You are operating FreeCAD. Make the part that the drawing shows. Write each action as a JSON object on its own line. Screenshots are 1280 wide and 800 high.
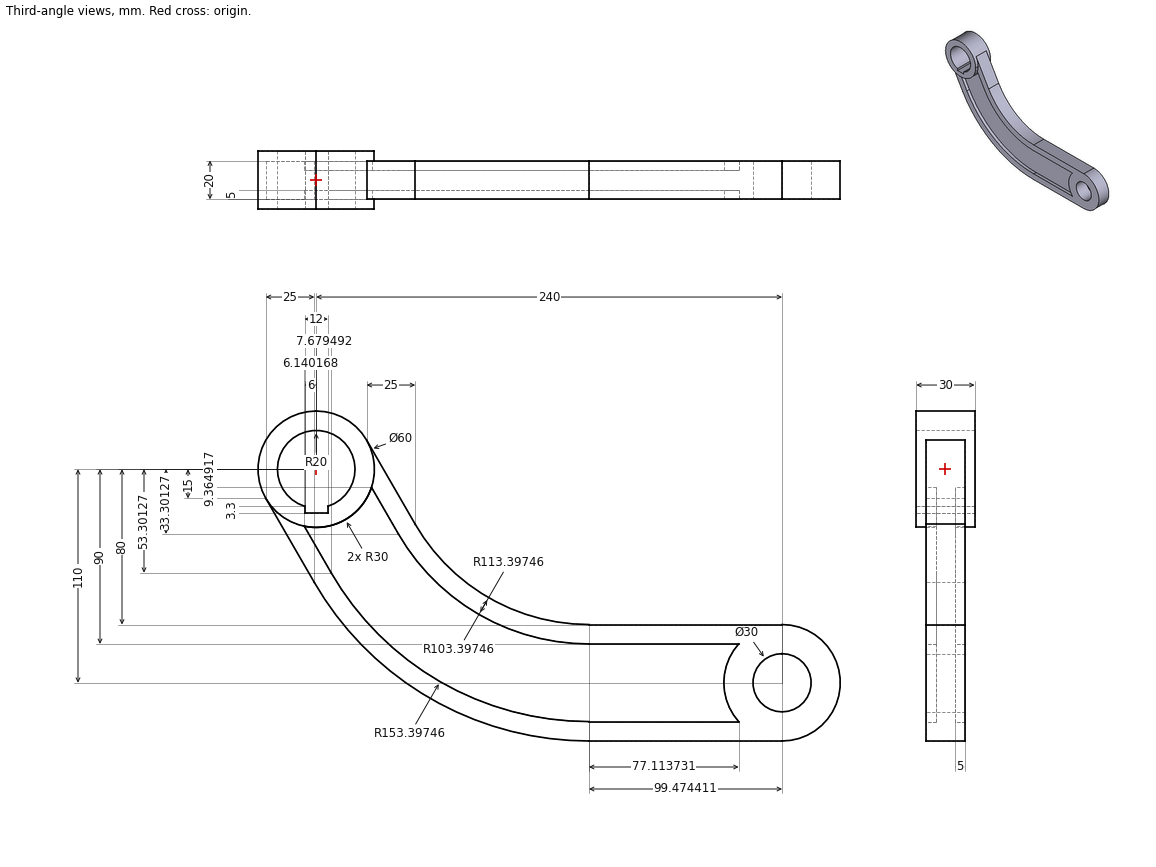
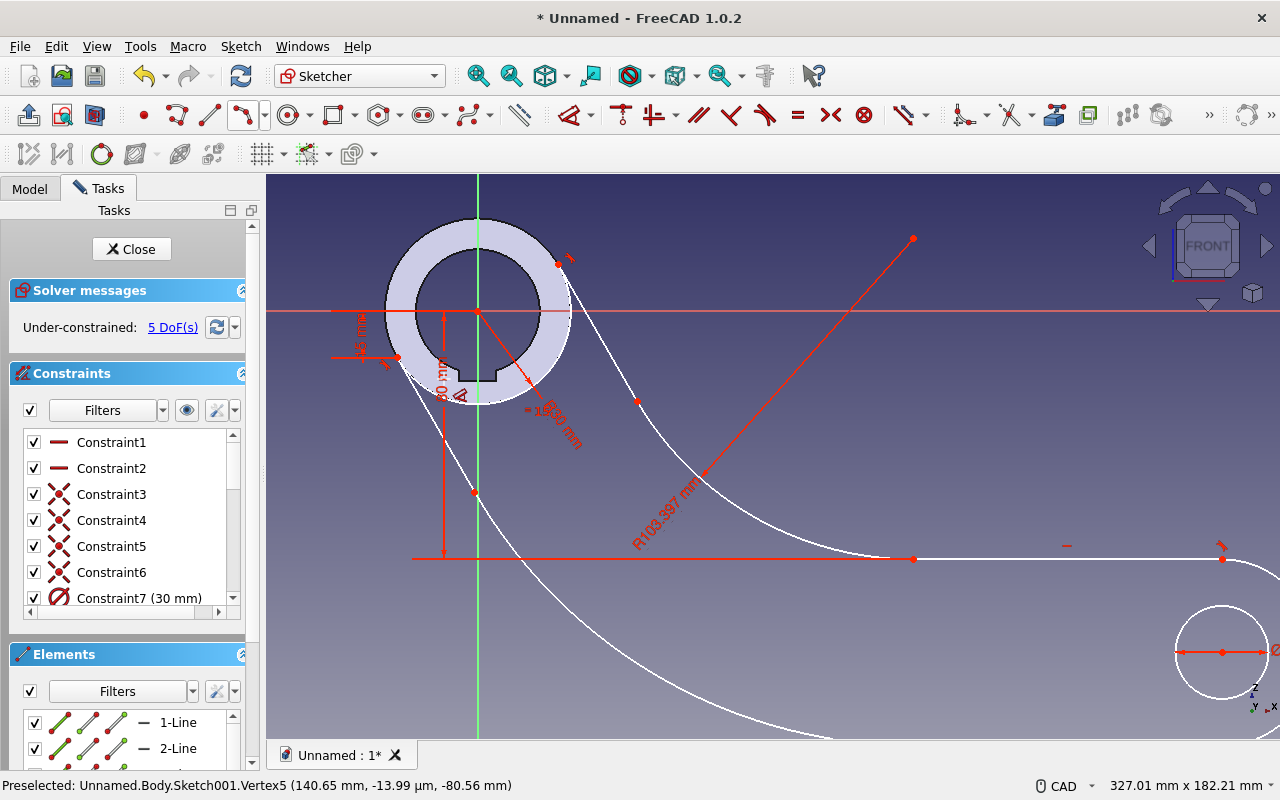
{"action": "left_click", "coordinate": [452, 452]}
{"action": "left_click", "coordinate": [436, 526]}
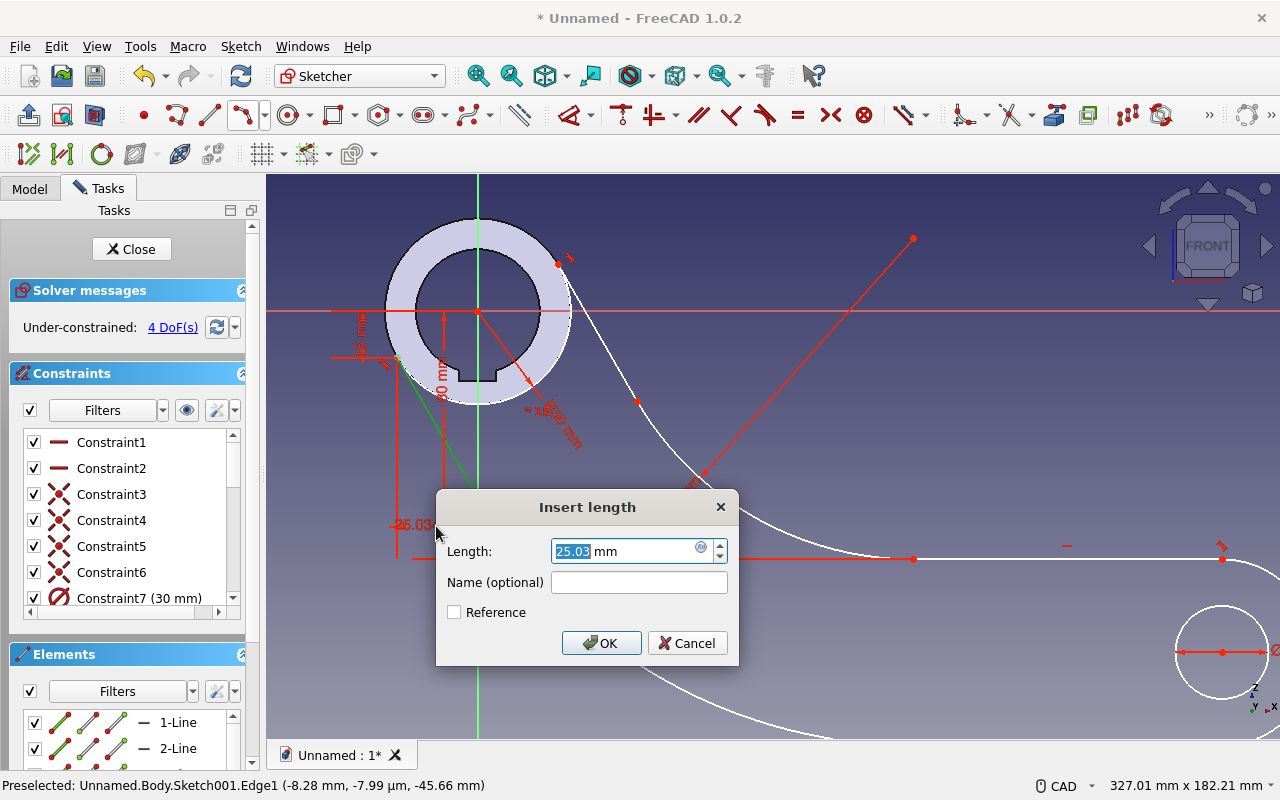
{"action": "type", "text": "25"}
{"action": "key", "text": "Return"}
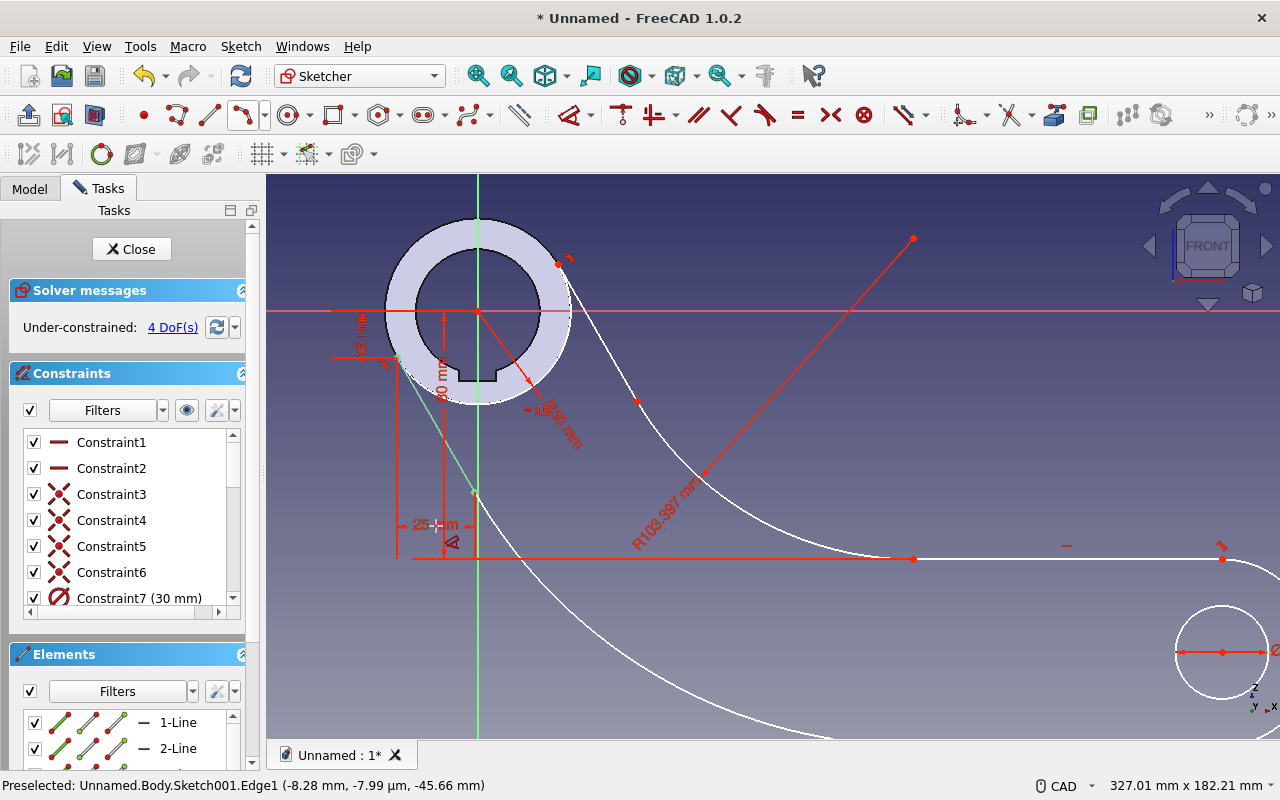
{"action": "left_click", "coordinate": [614, 360]}
{"action": "left_click", "coordinate": [598, 231]}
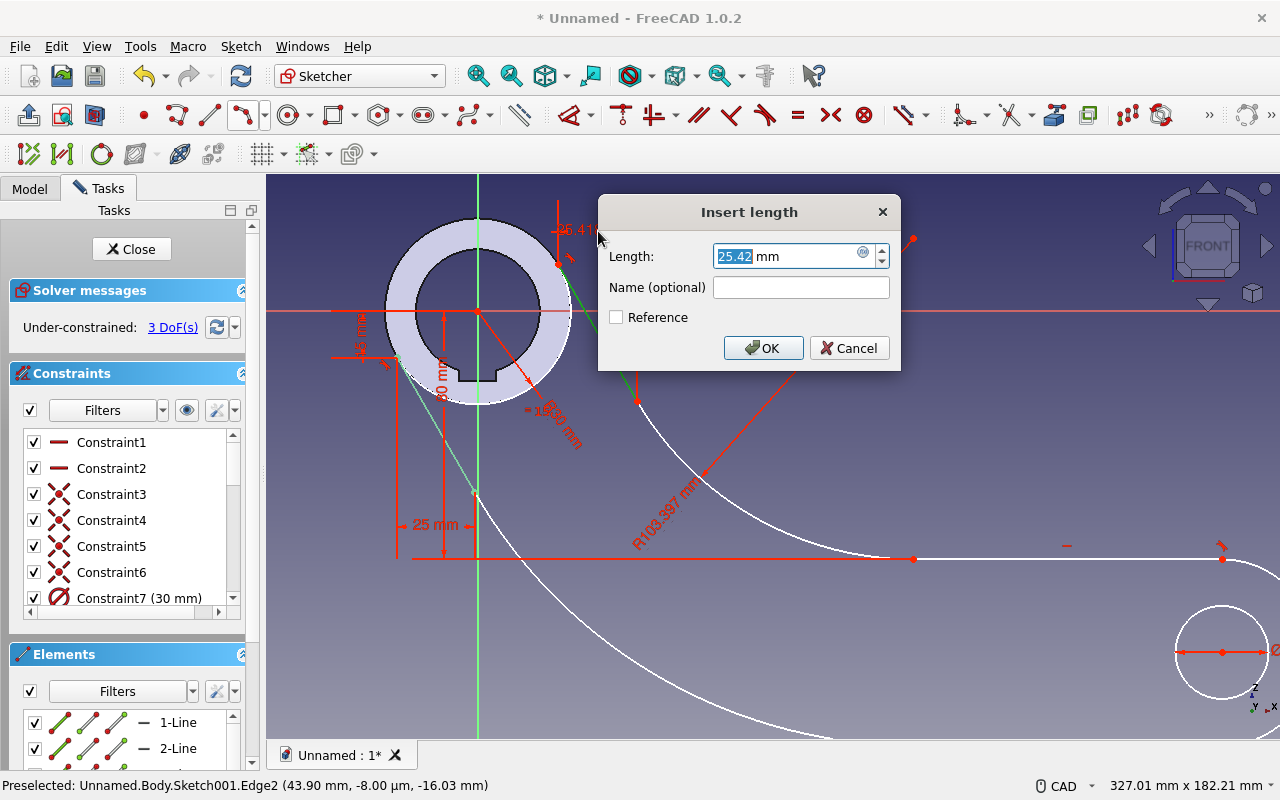
{"action": "type", "text": "25"}
{"action": "key", "text": "Return"}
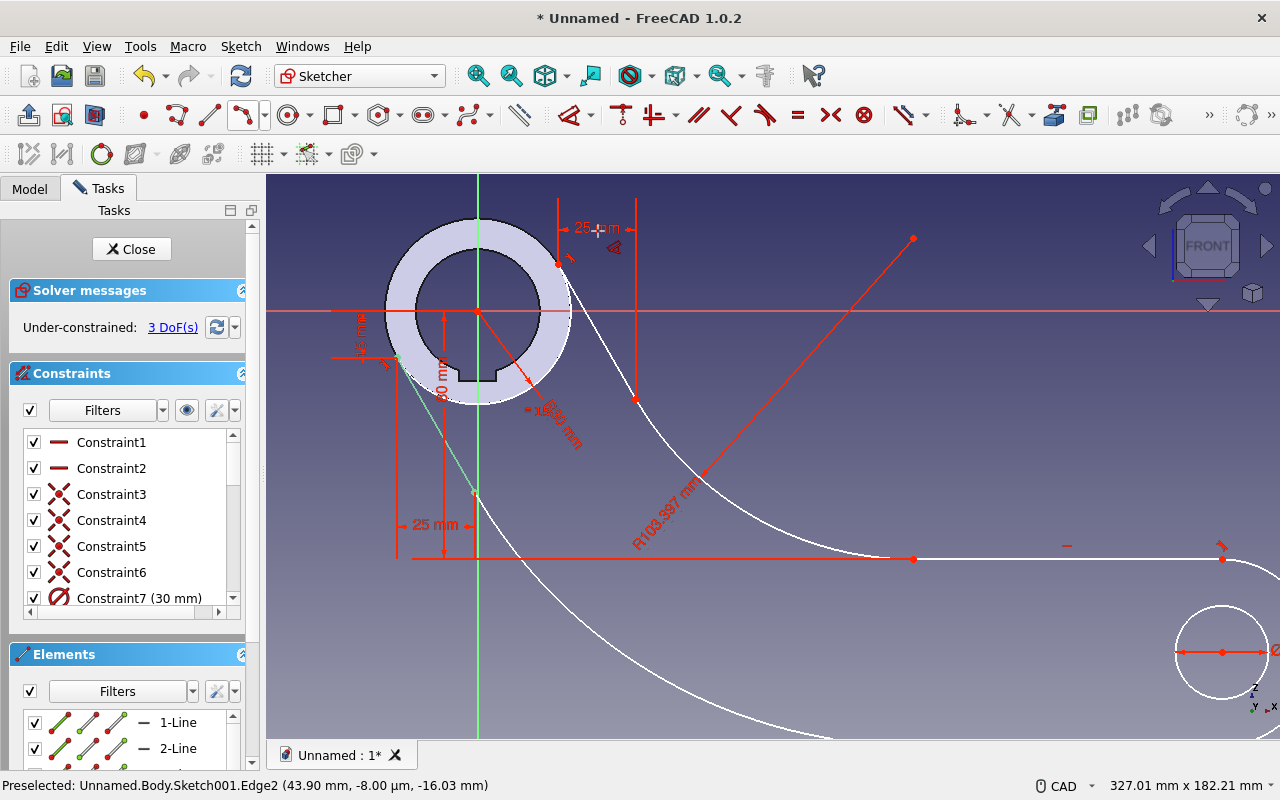
{"action": "scroll", "coordinate": [396, 358], "scroll_direction": "down", "scroll_amount": 2}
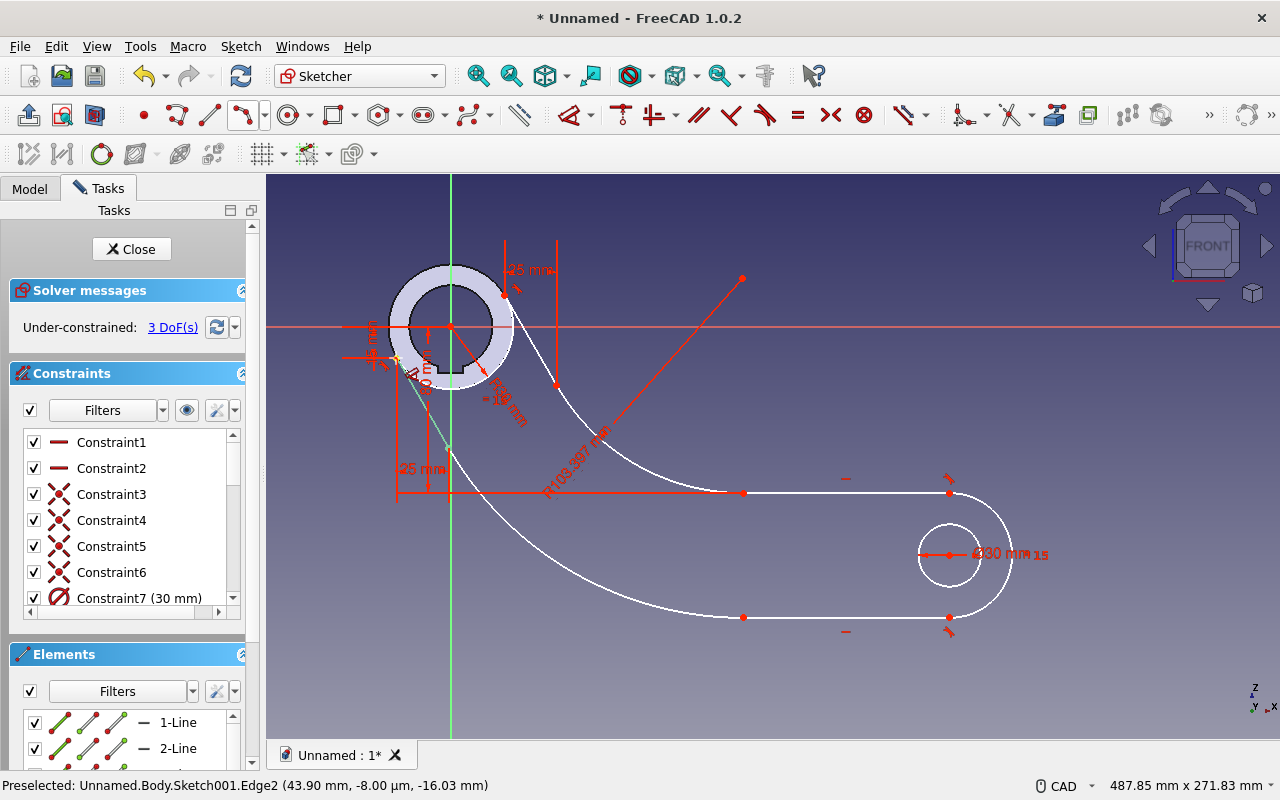
{"action": "left_click", "coordinate": [950, 555]}
{"action": "left_click", "coordinate": [700, 293]}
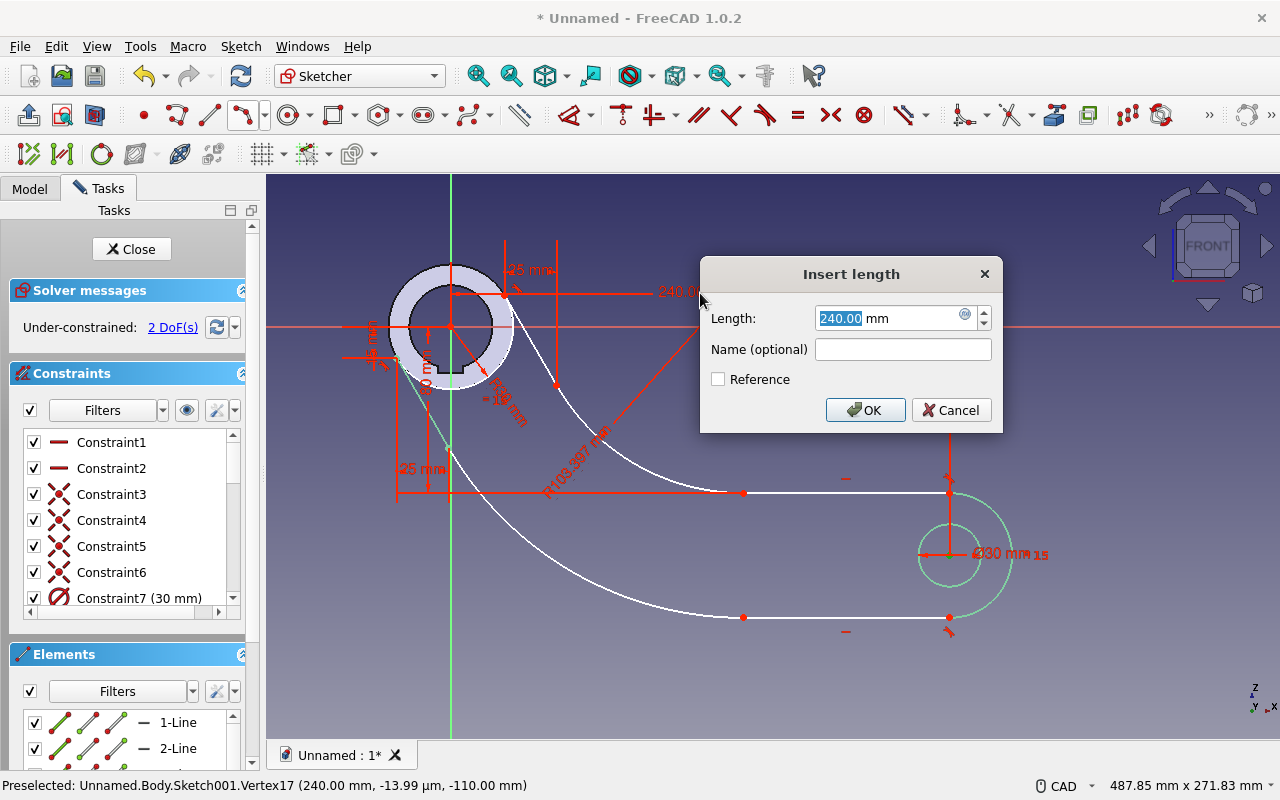
{"action": "type", "text": "240"}
{"action": "key", "text": "Return"}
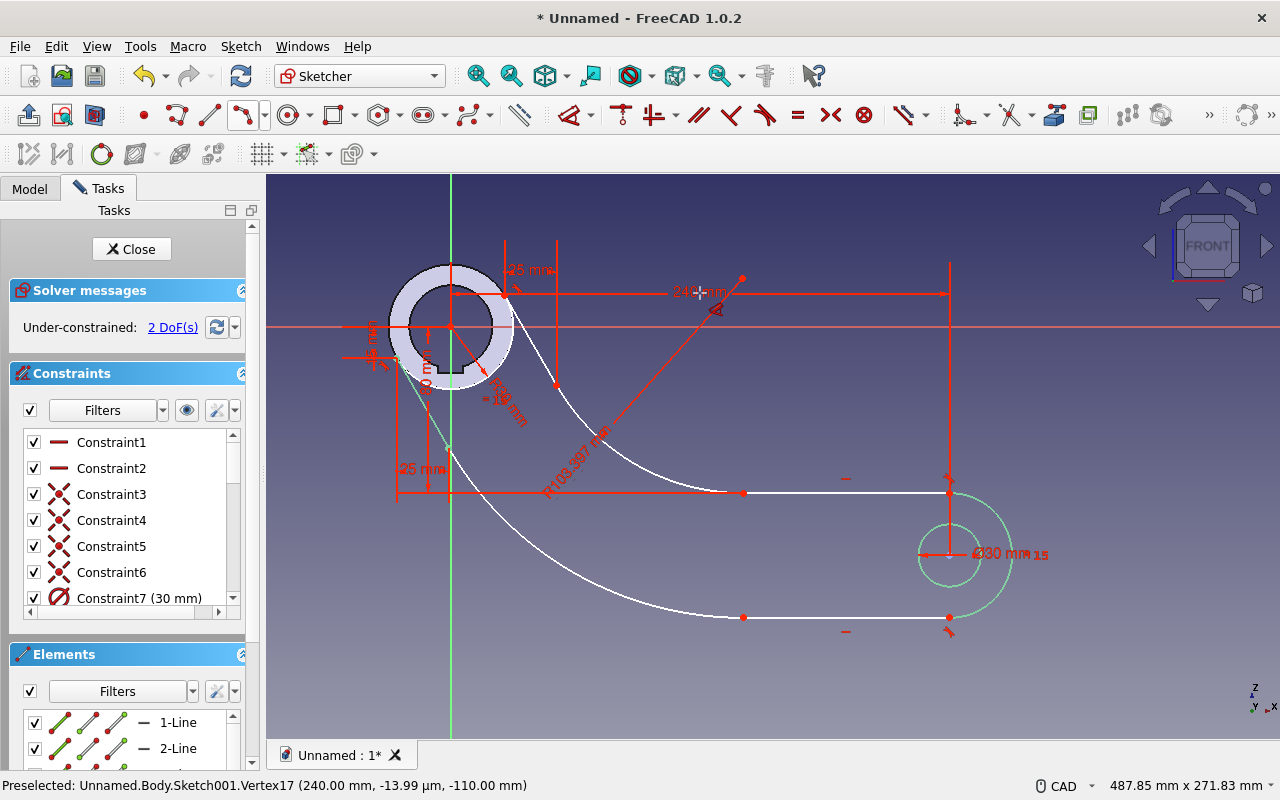
{"action": "left_click", "coordinate": [805, 493]}
{"action": "left_click", "coordinate": [846, 527]}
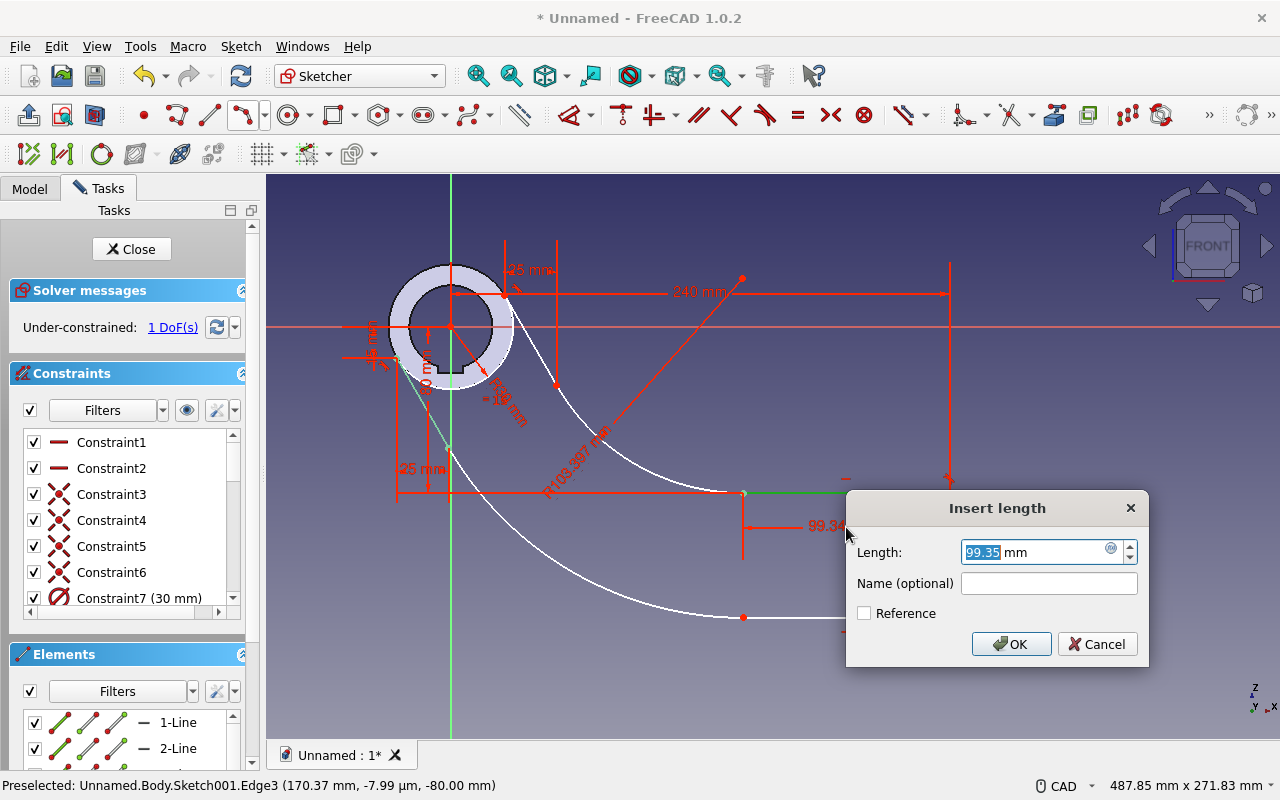
{"action": "type", "text": "99.474411"}
{"action": "key", "text": "Return"}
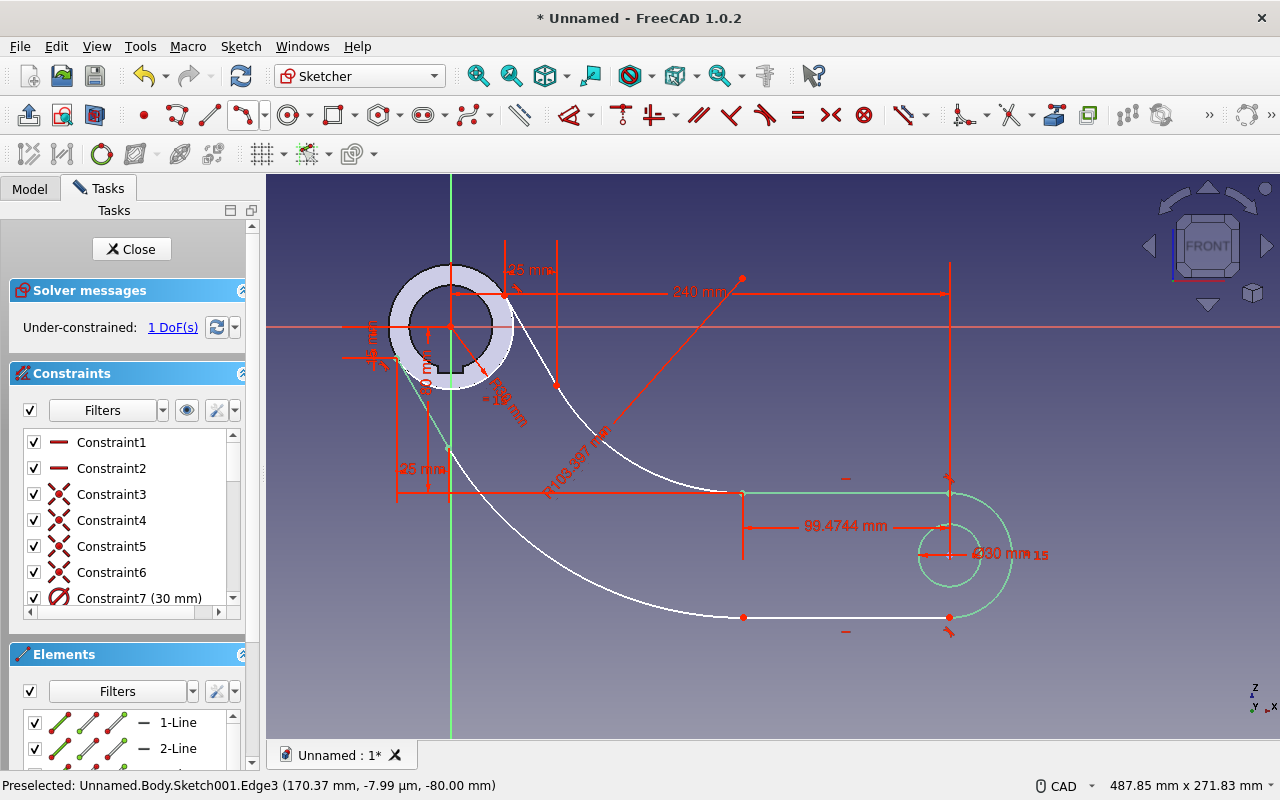
{"action": "left_click", "coordinate": [888, 618]}
{"action": "left_click", "coordinate": [846, 652]}